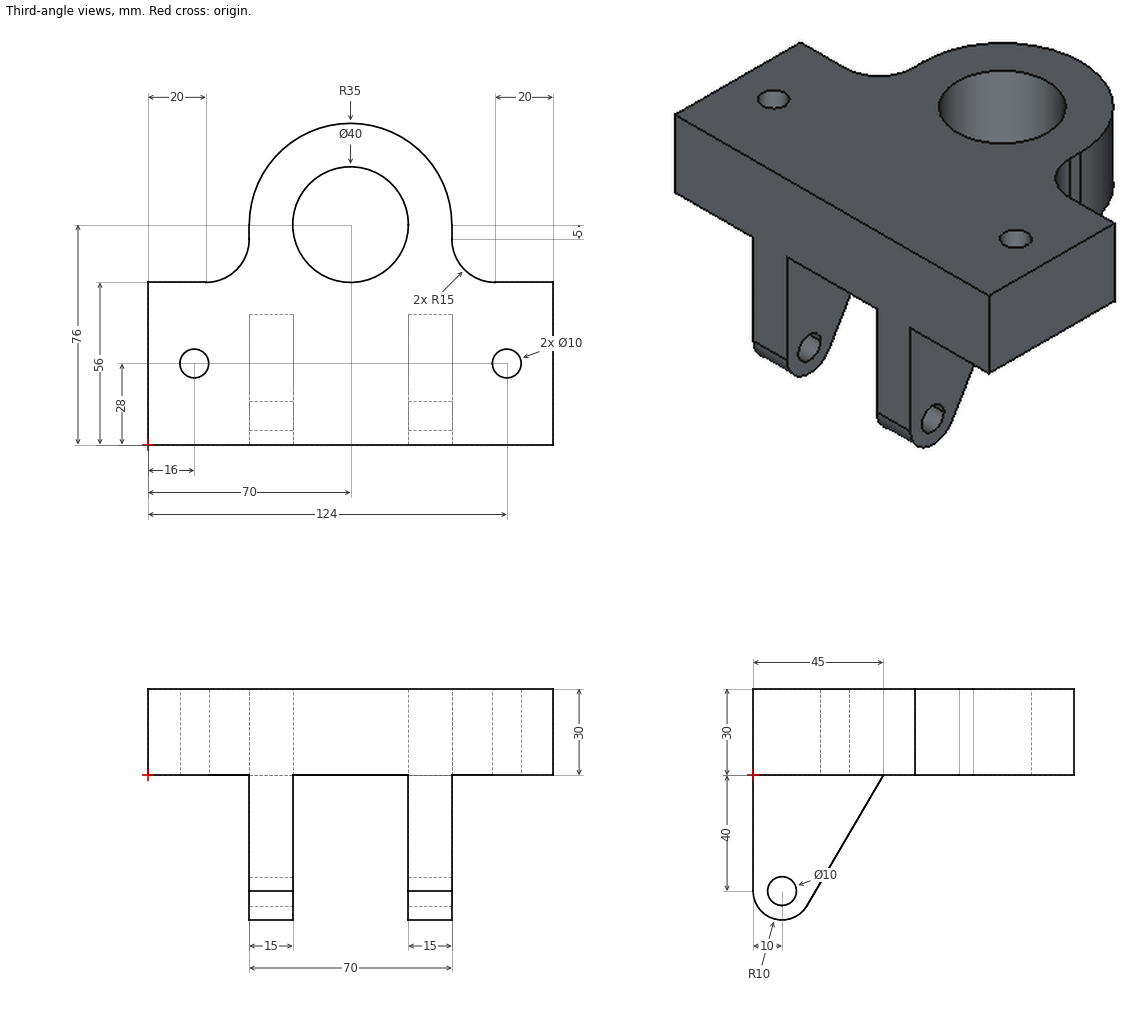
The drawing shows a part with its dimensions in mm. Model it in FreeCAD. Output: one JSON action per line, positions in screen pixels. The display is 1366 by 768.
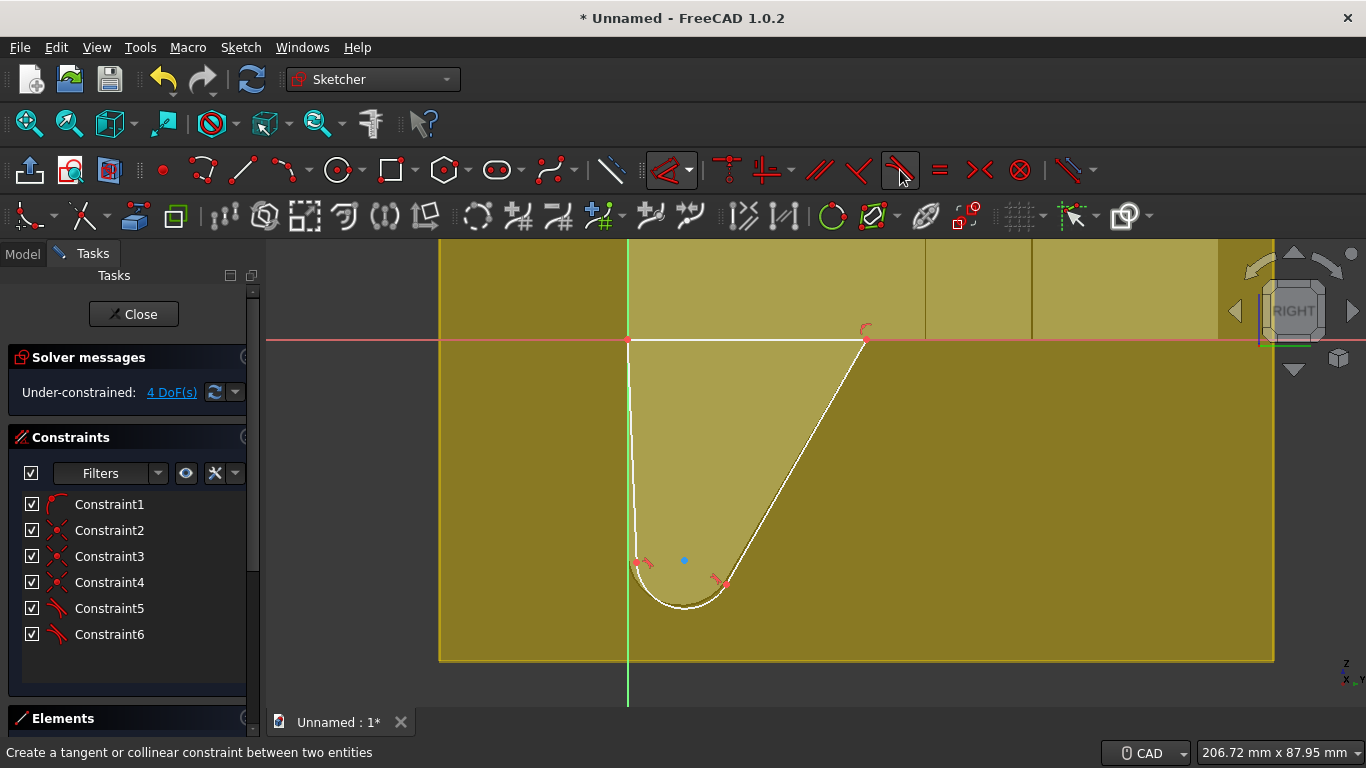
{"action": "left_click", "coordinate": [630, 407]}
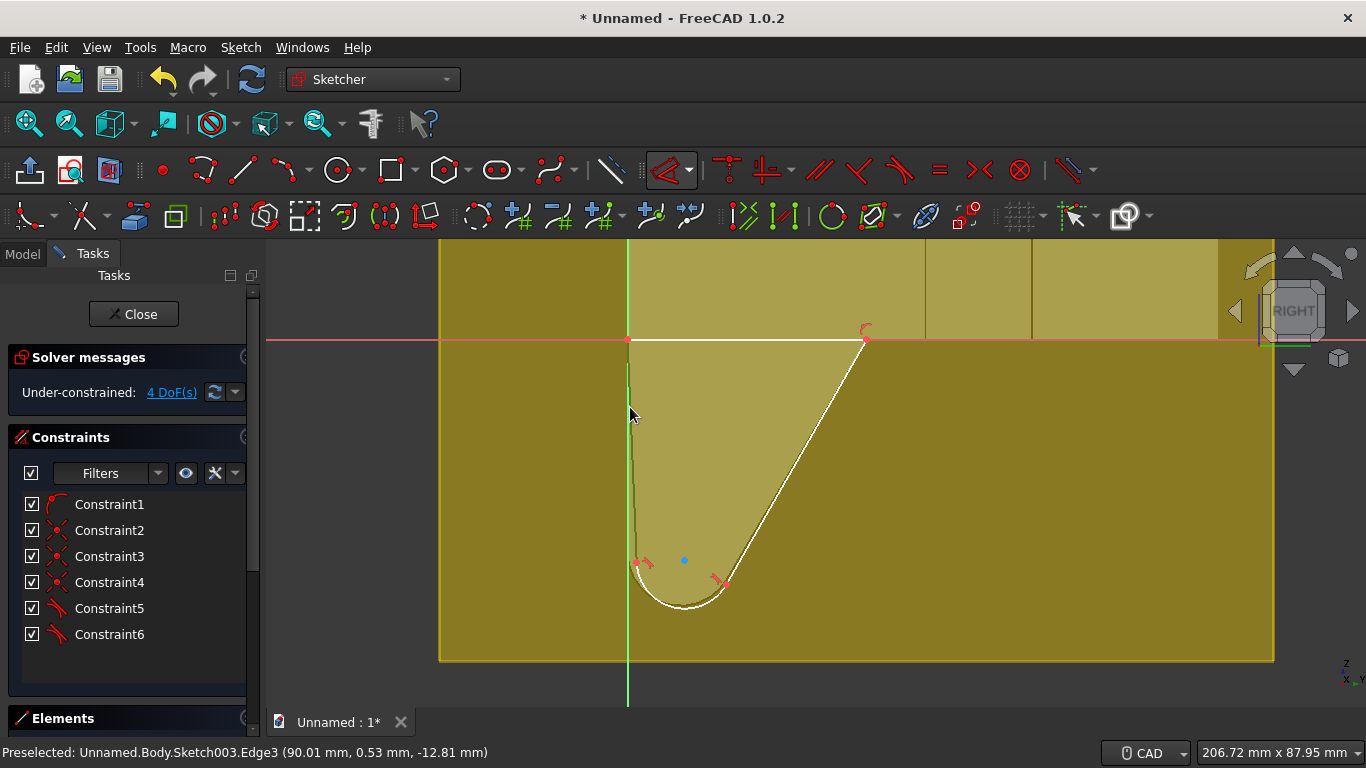
{"action": "left_click", "coordinate": [794, 170]}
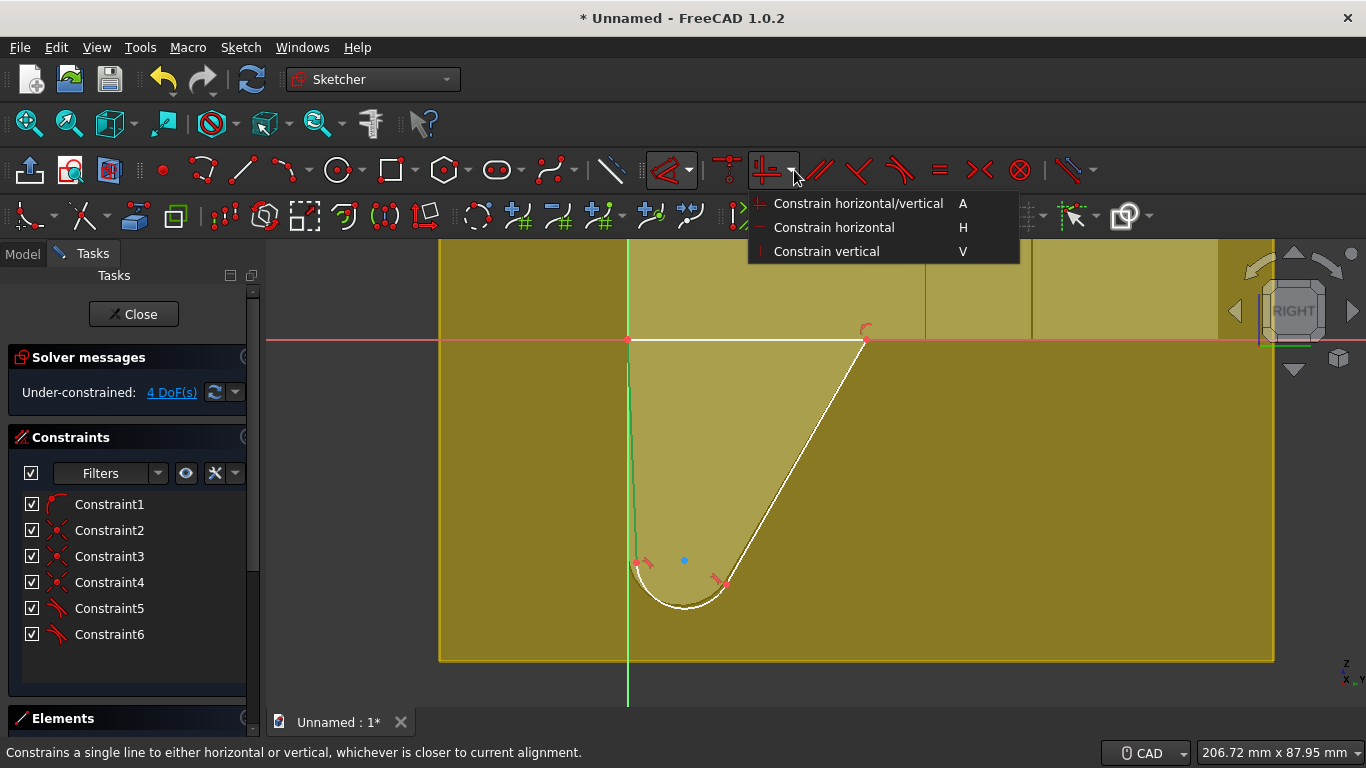
{"action": "left_click", "coordinate": [884, 251]}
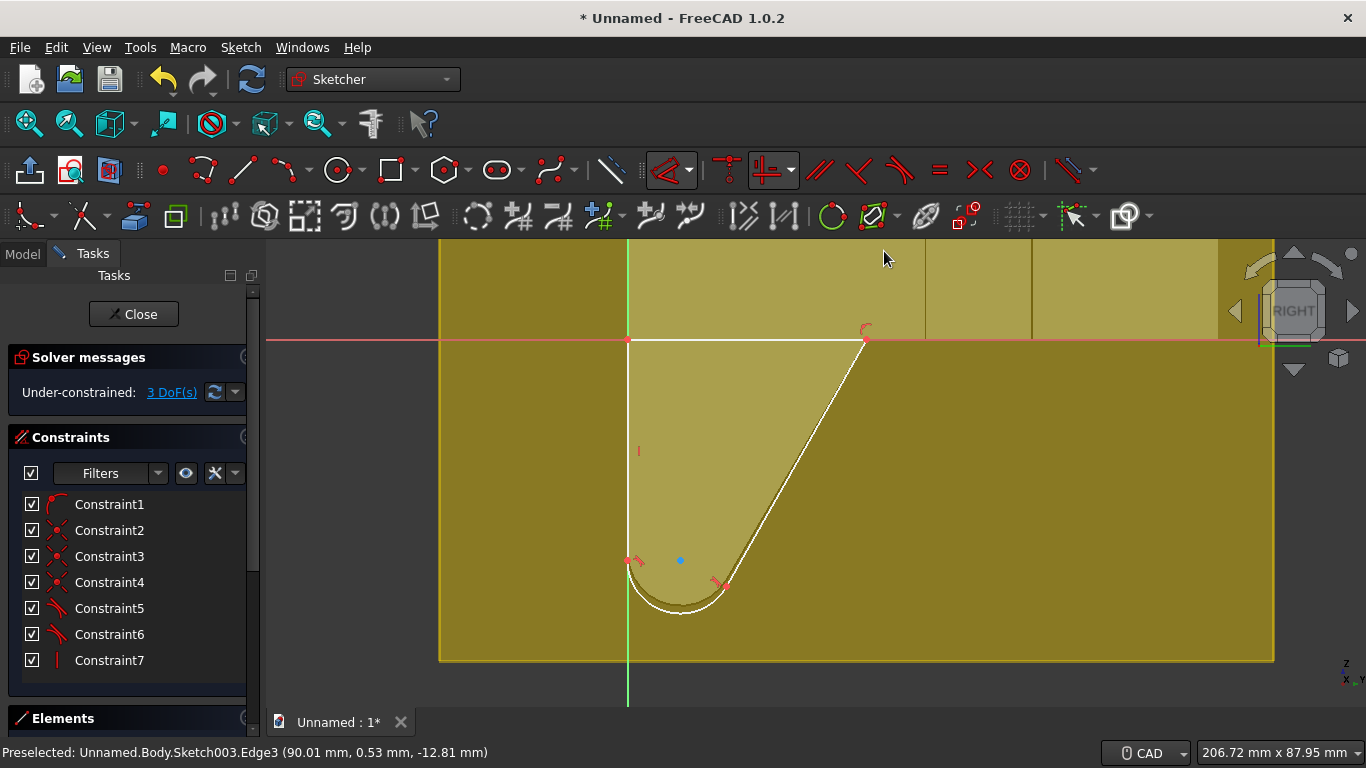
{"action": "left_click", "coordinate": [643, 598]}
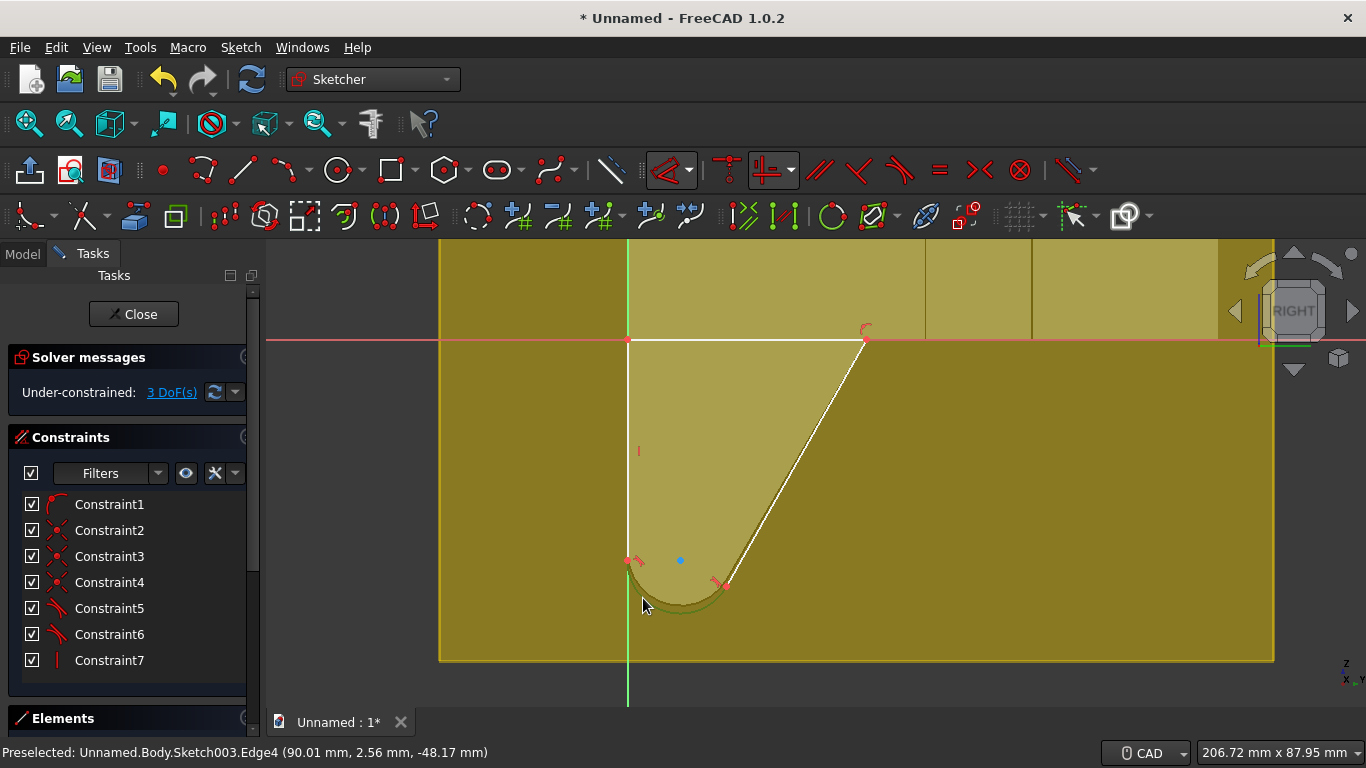
{"action": "key", "text": "k r"}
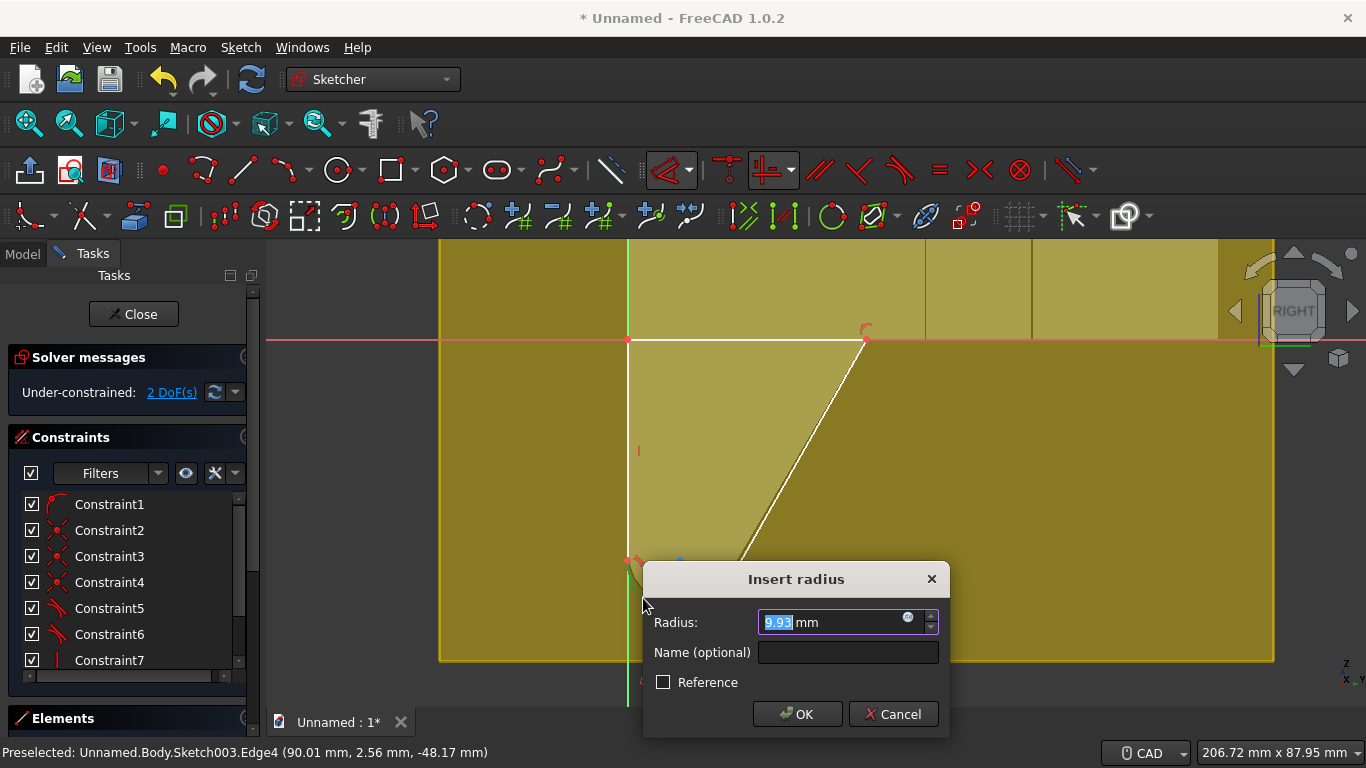
{"action": "type", "text": "10"}
{"action": "key", "text": "Return"}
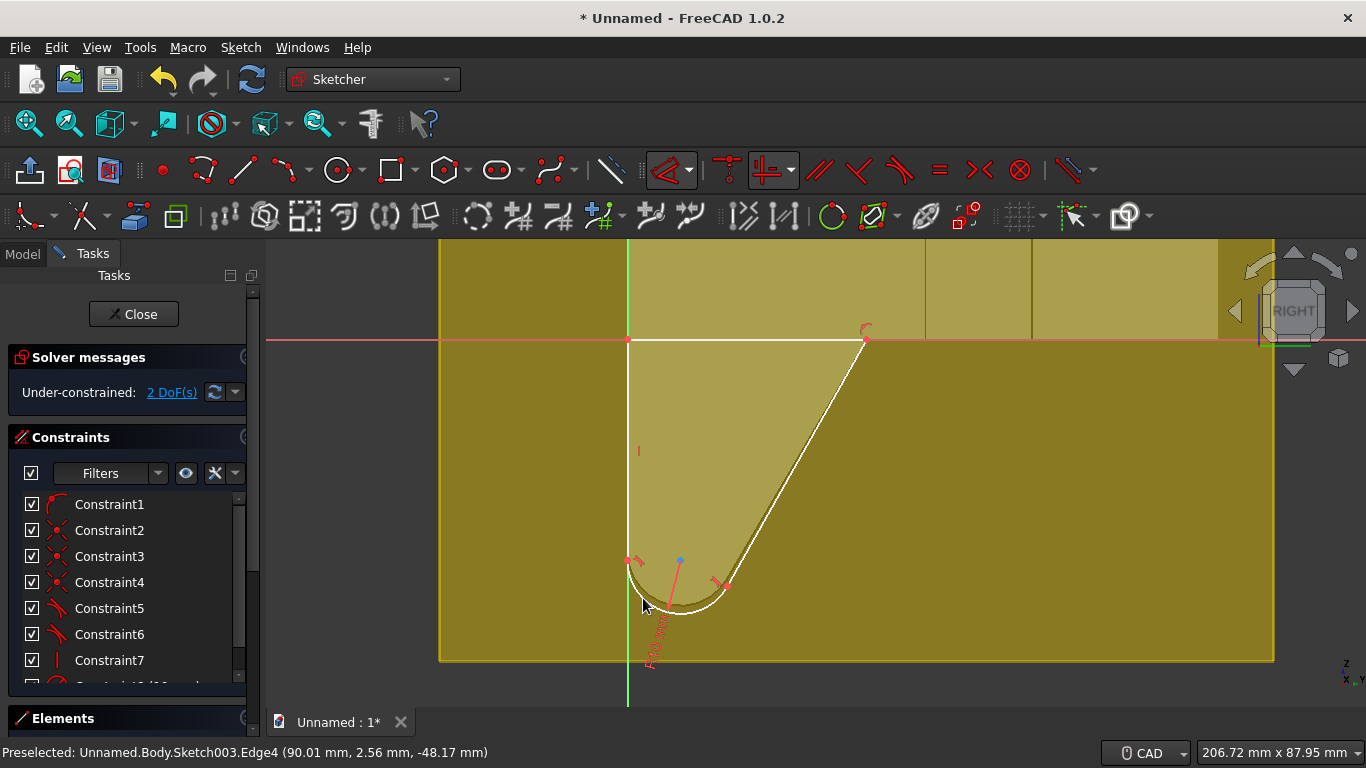
{"action": "left_click", "coordinate": [795, 340]}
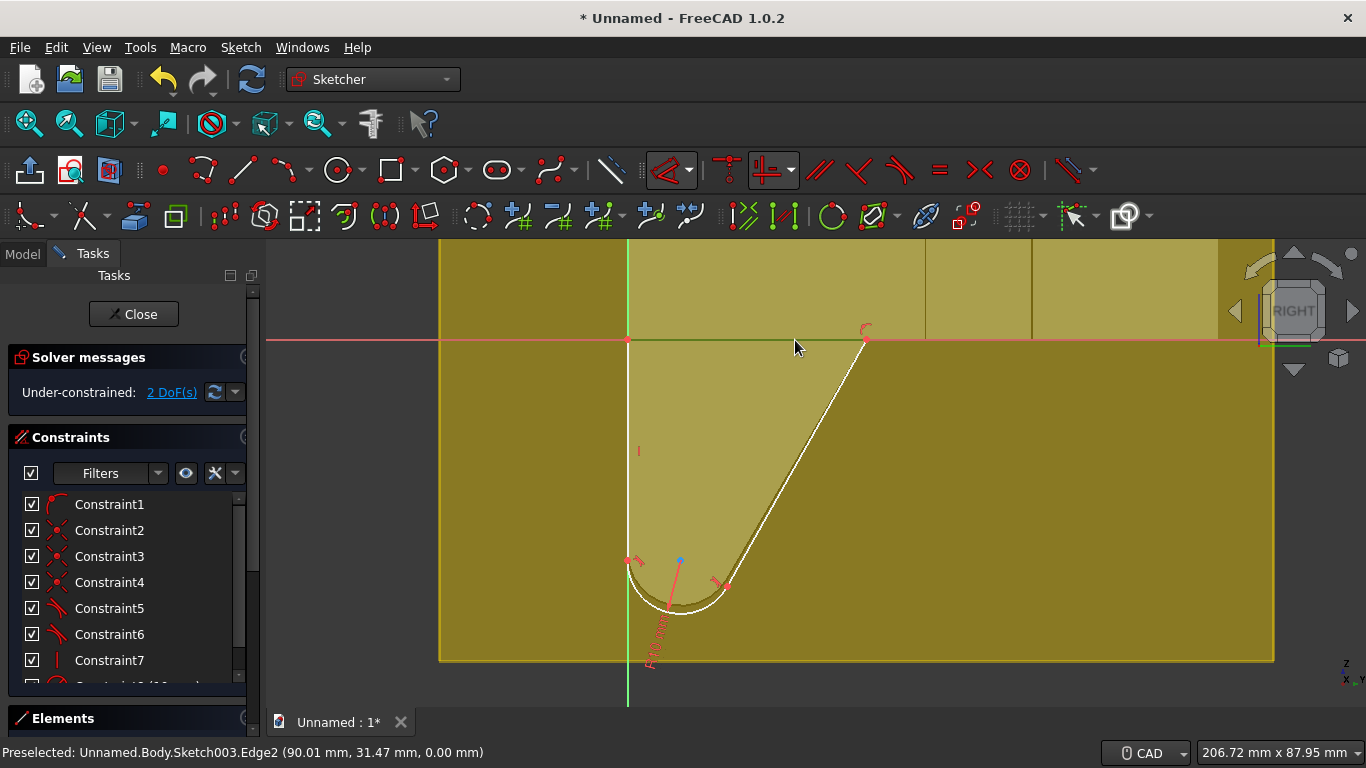
{"action": "left_click", "coordinate": [692, 170]}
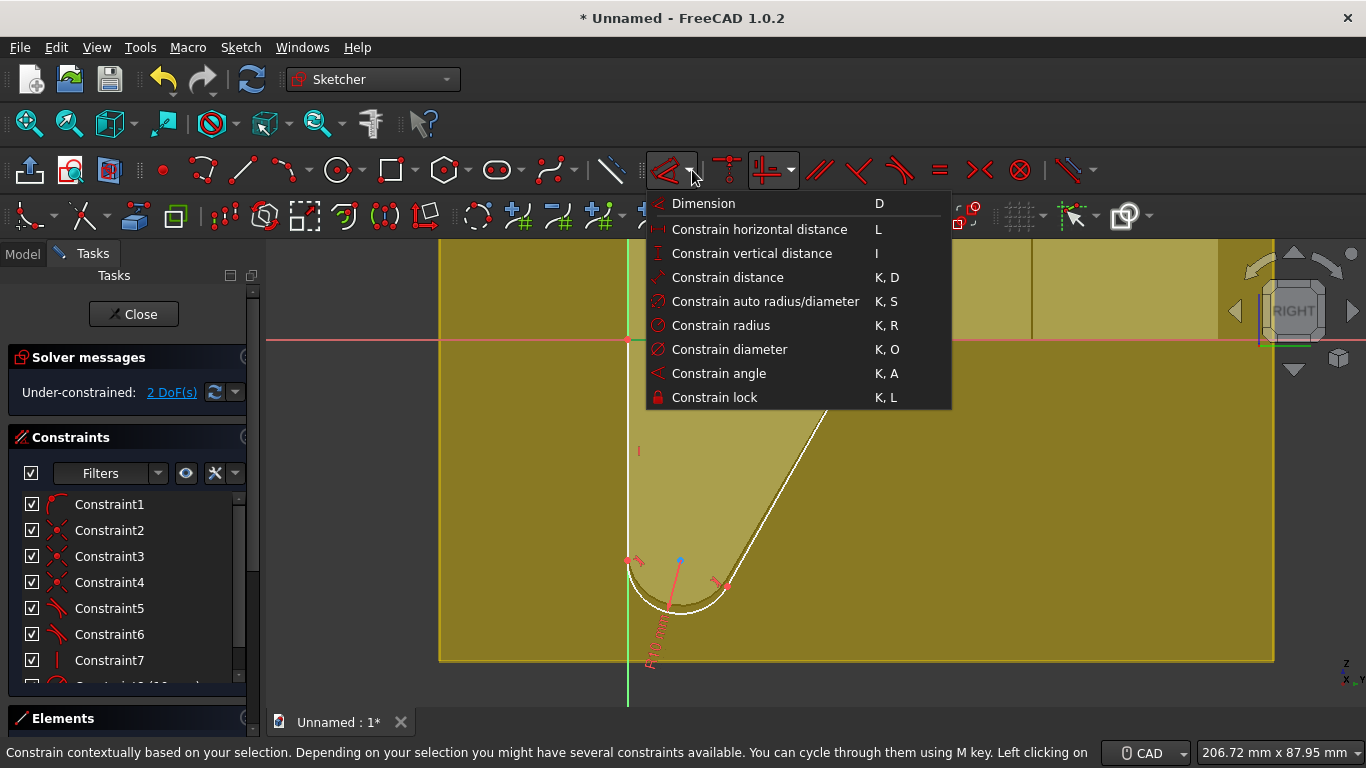
{"action": "left_click", "coordinate": [799, 229]}